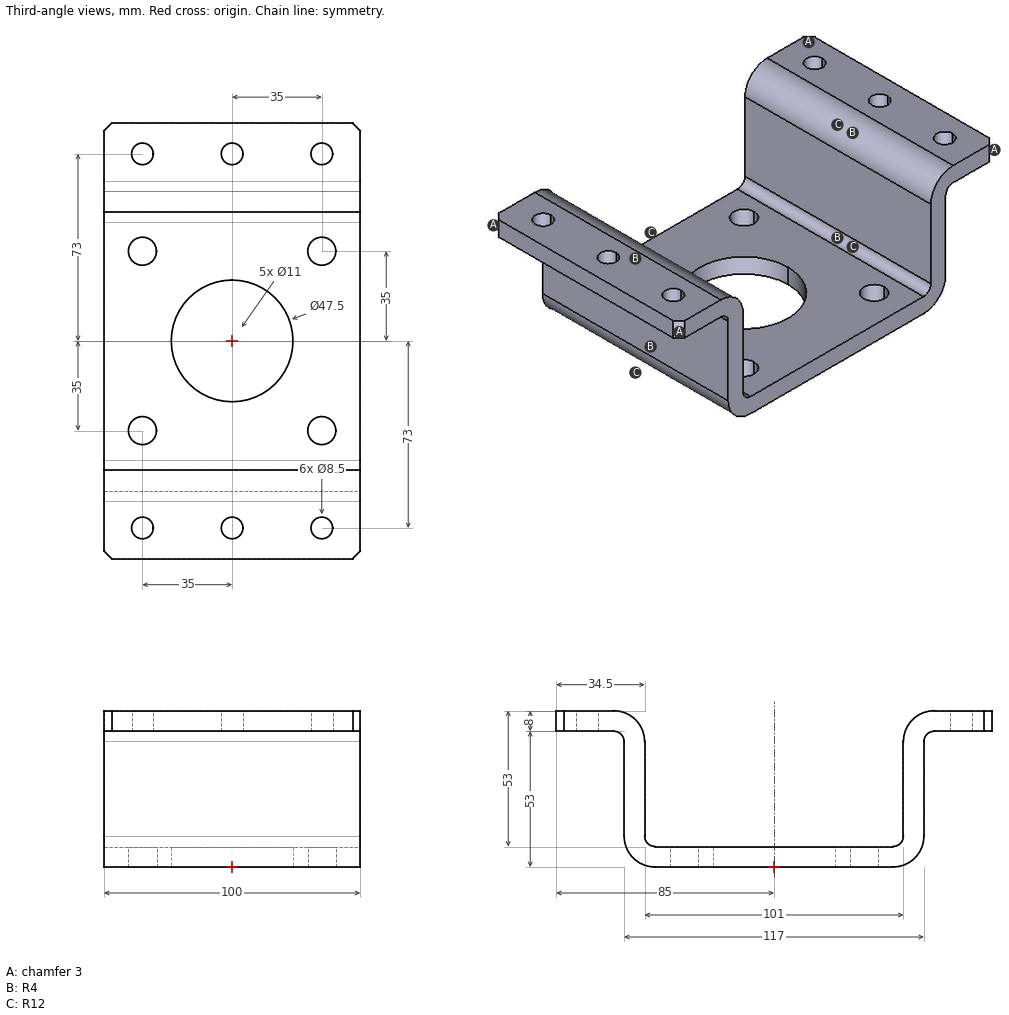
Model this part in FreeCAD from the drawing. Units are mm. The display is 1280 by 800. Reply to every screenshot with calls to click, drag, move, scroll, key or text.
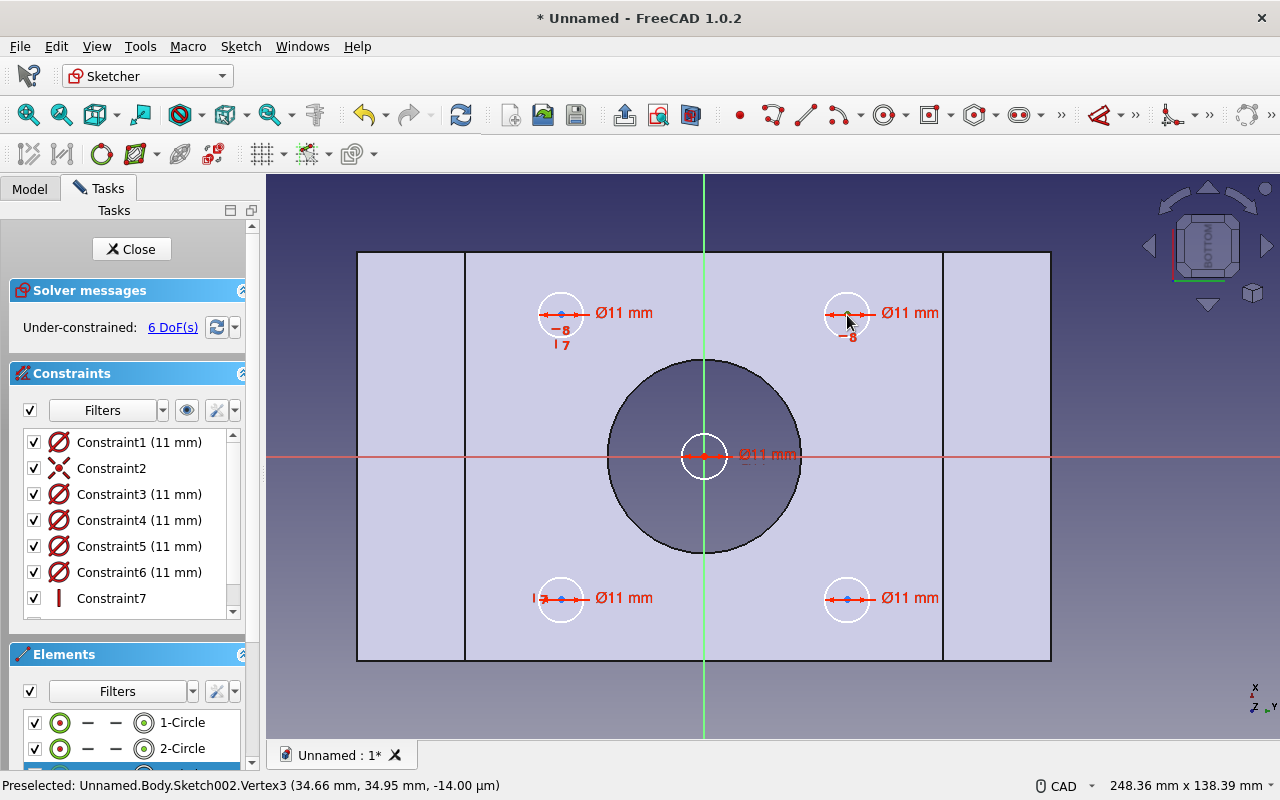
click(847, 600)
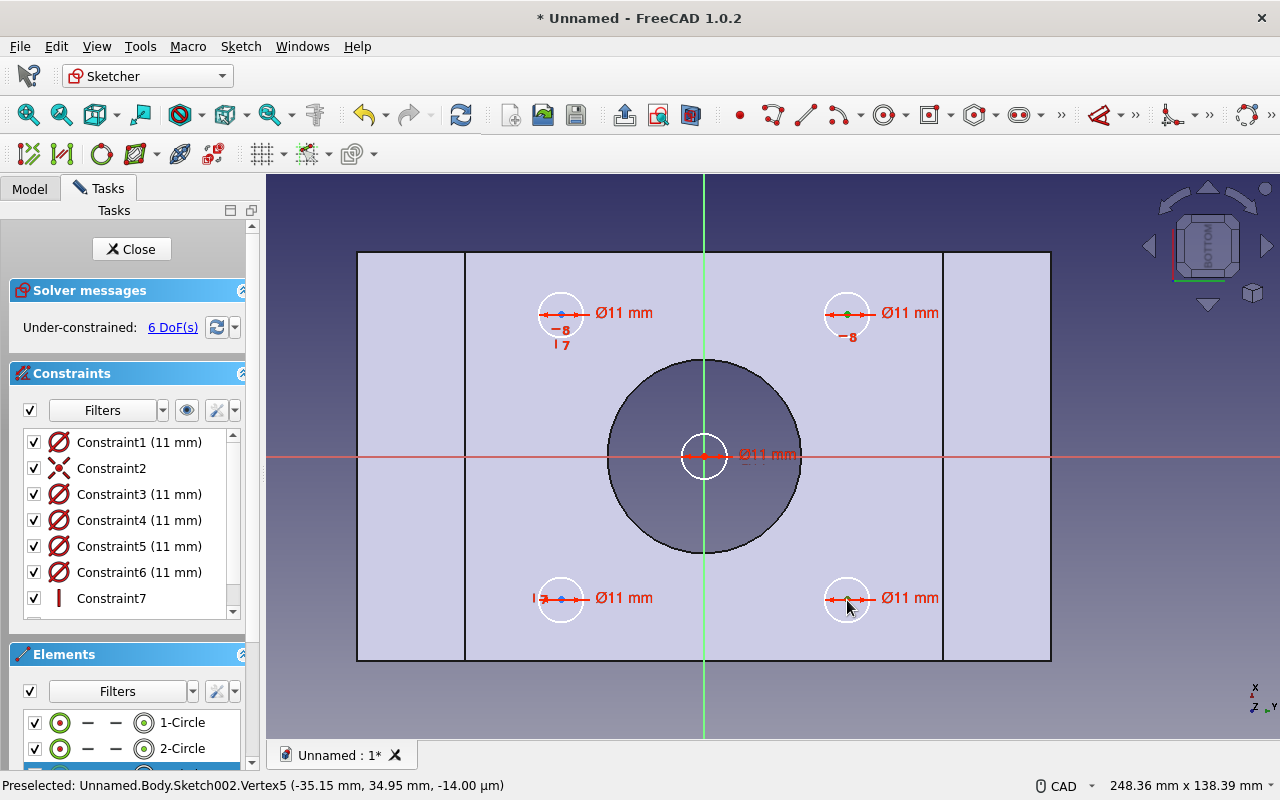
key(v)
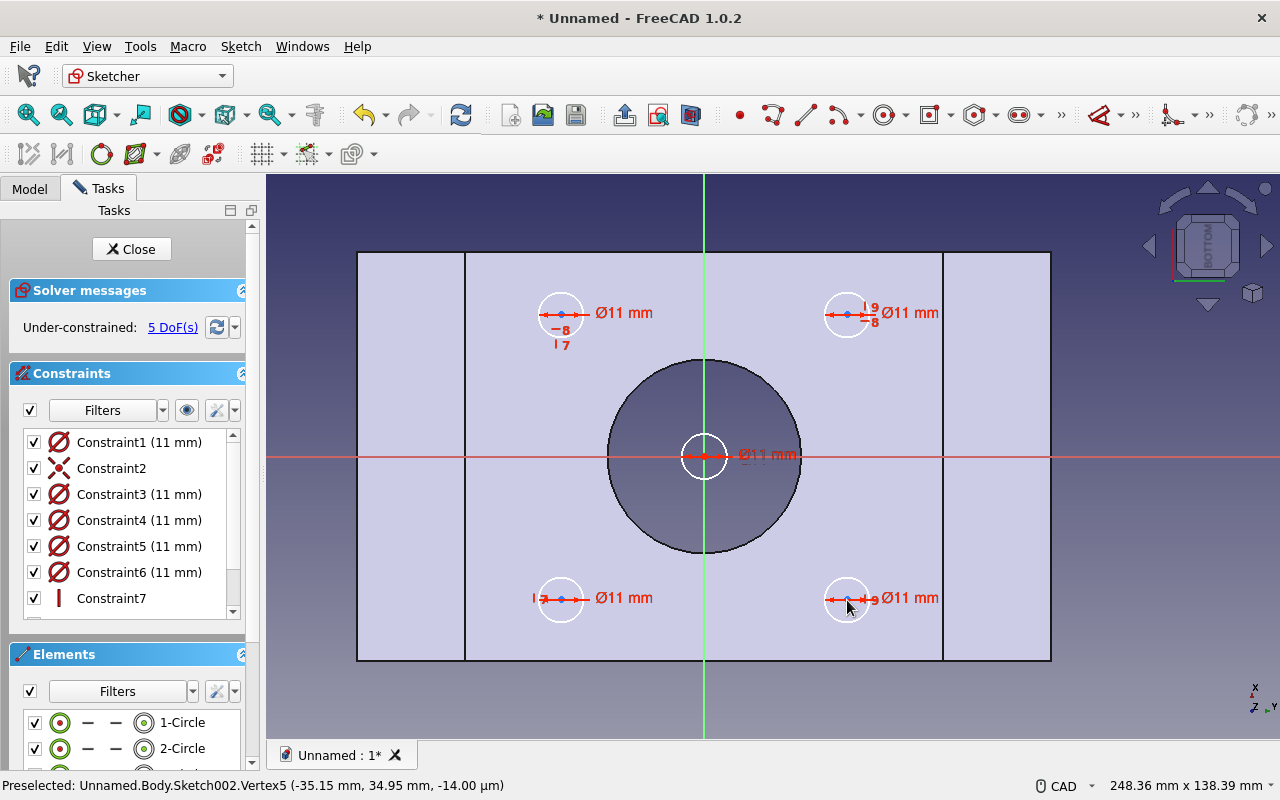
click(561, 600)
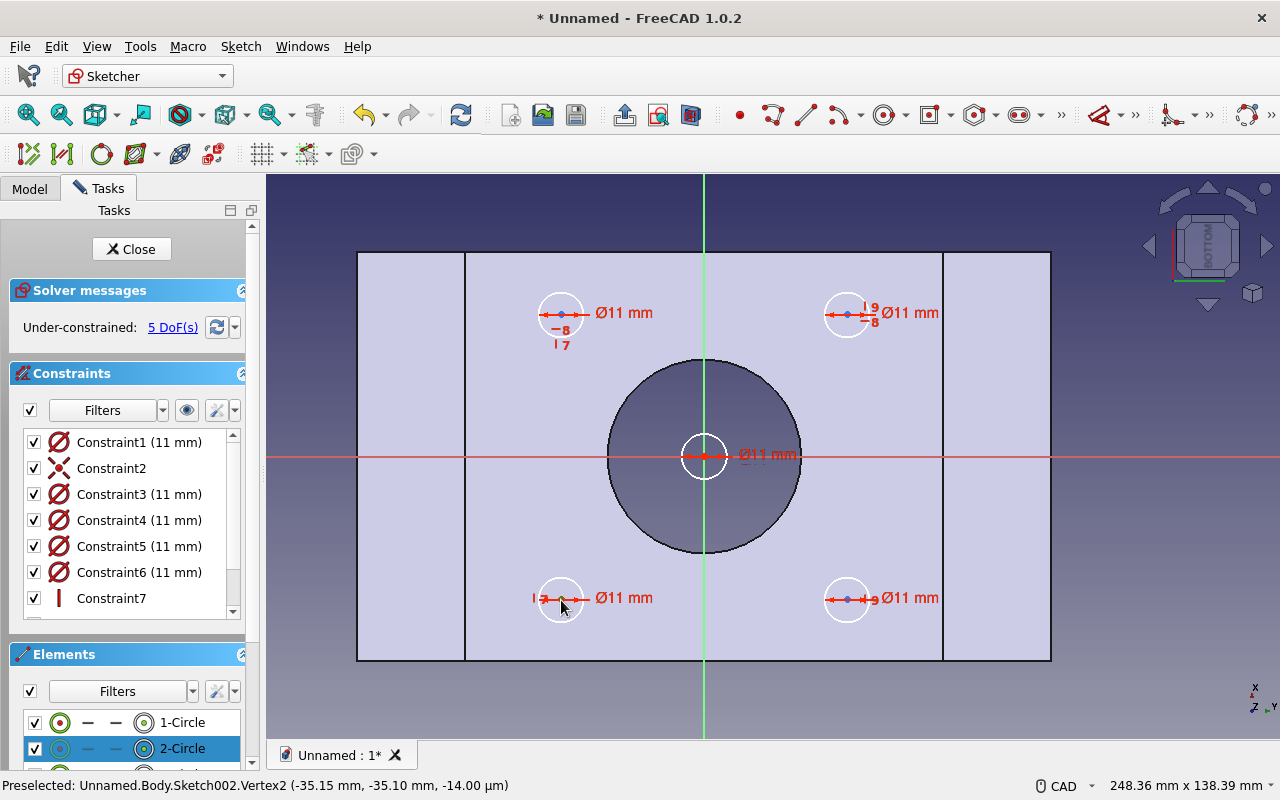
click(847, 600)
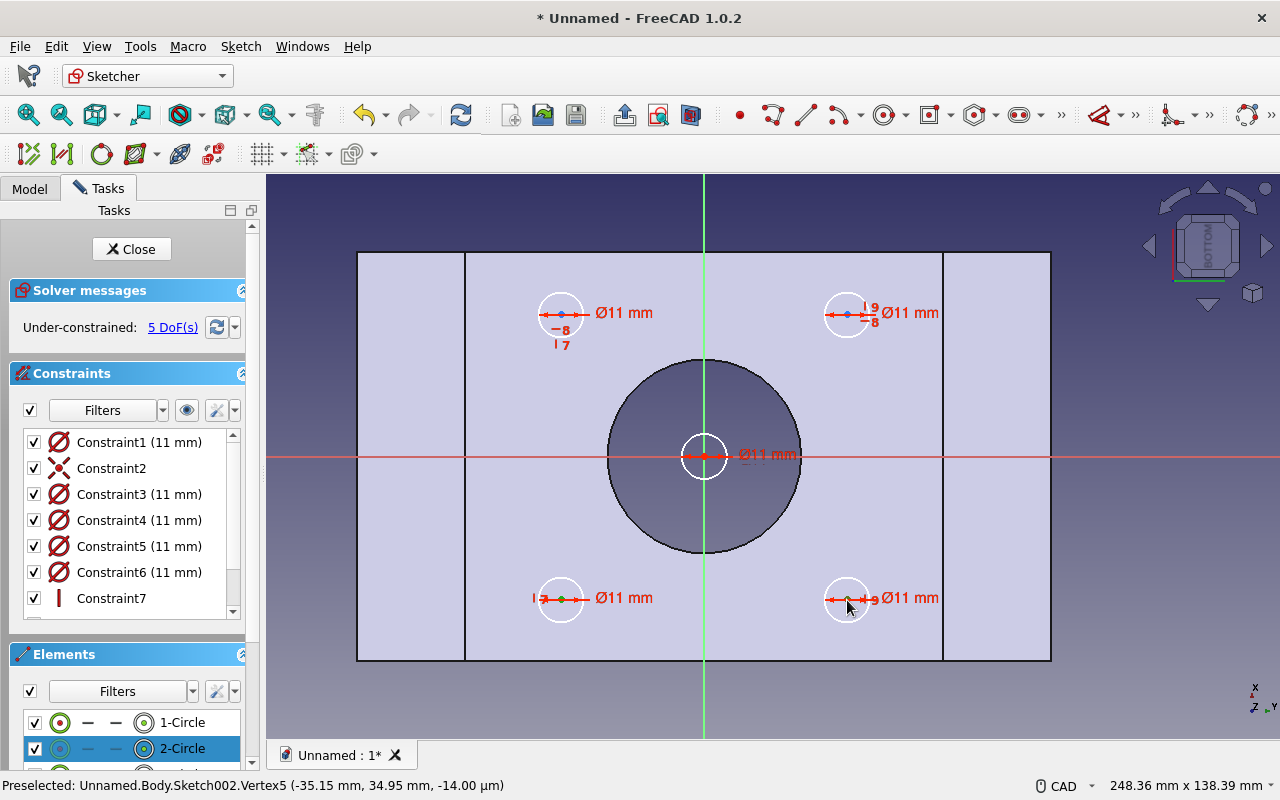
key(h)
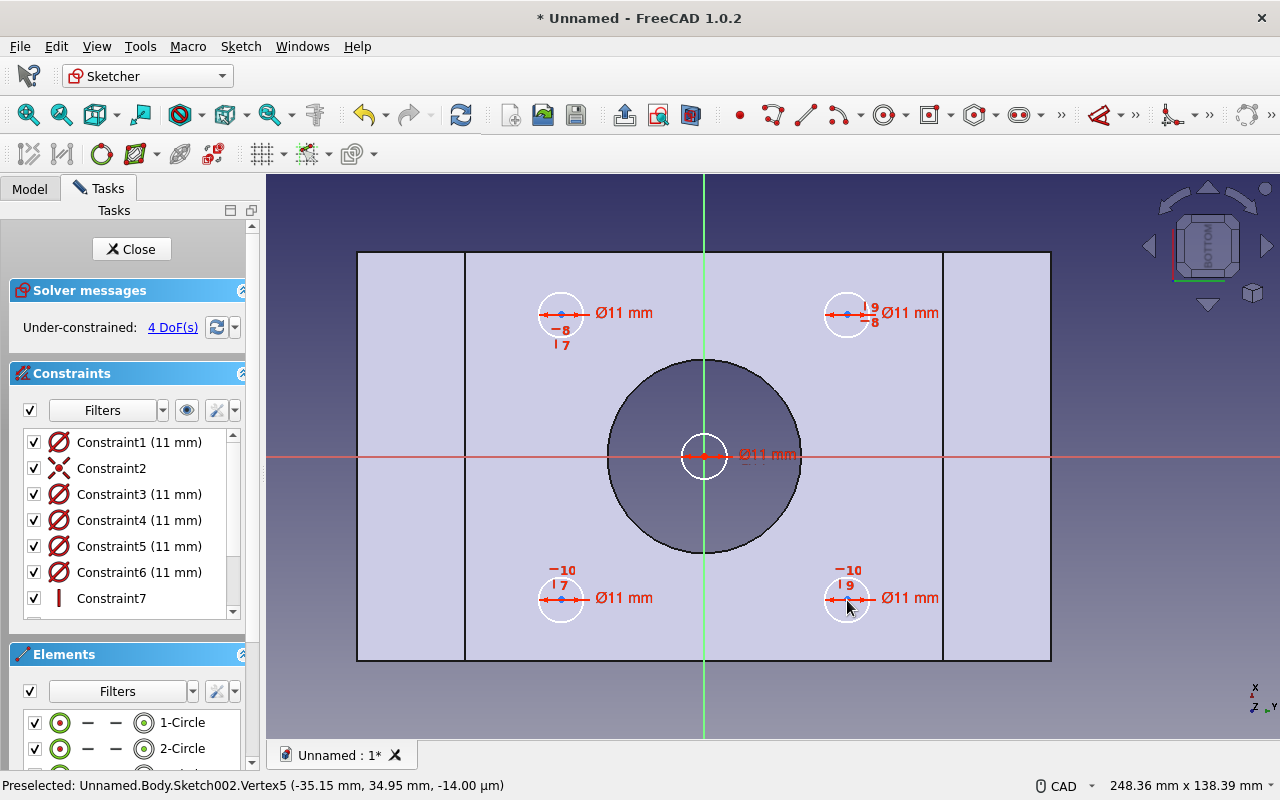
key(d)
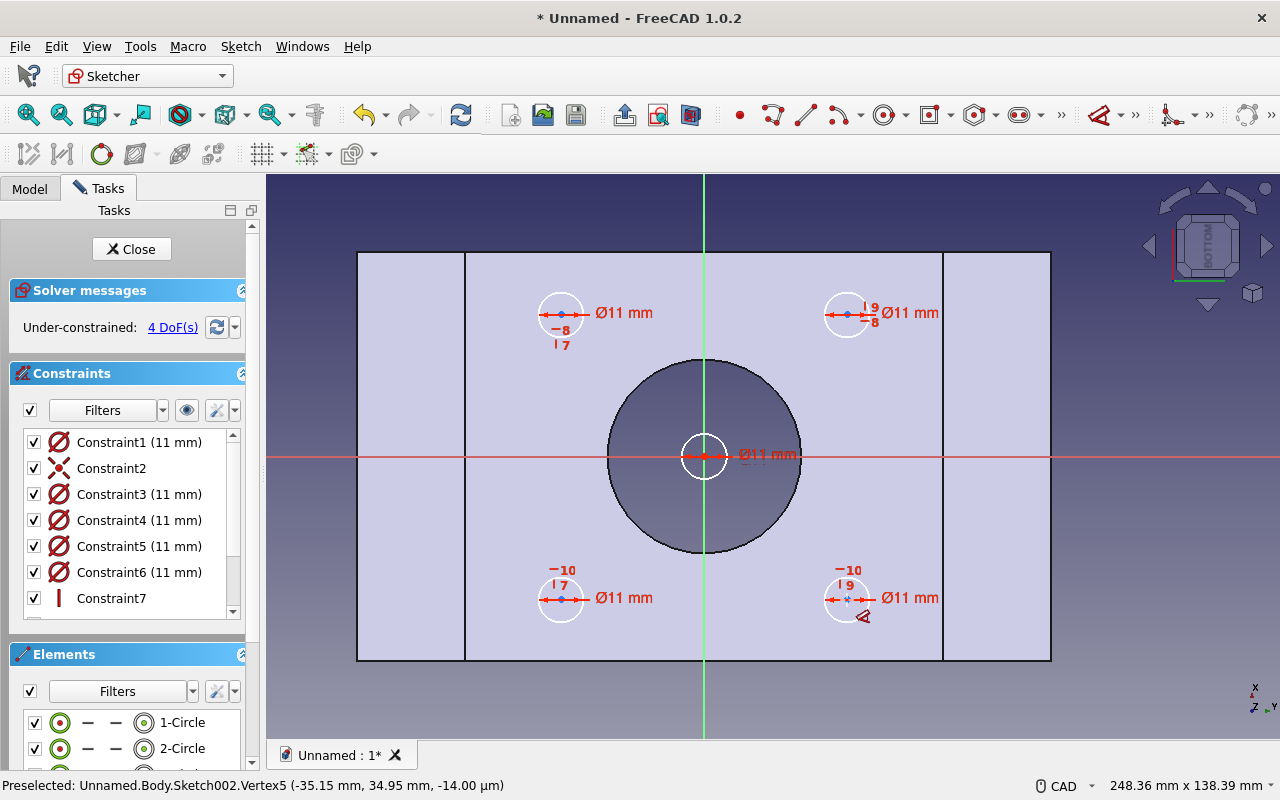
click(561, 600)
click(633, 634)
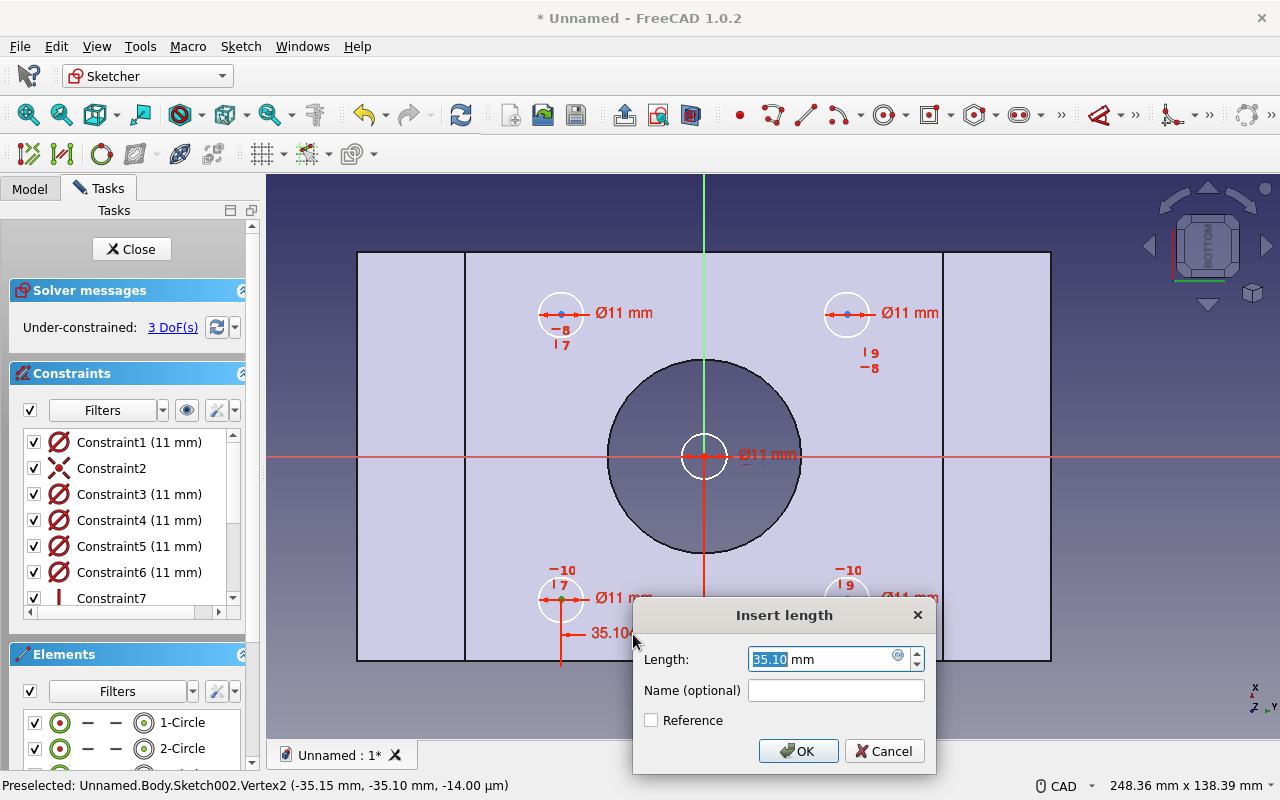
text(35)
key(Return)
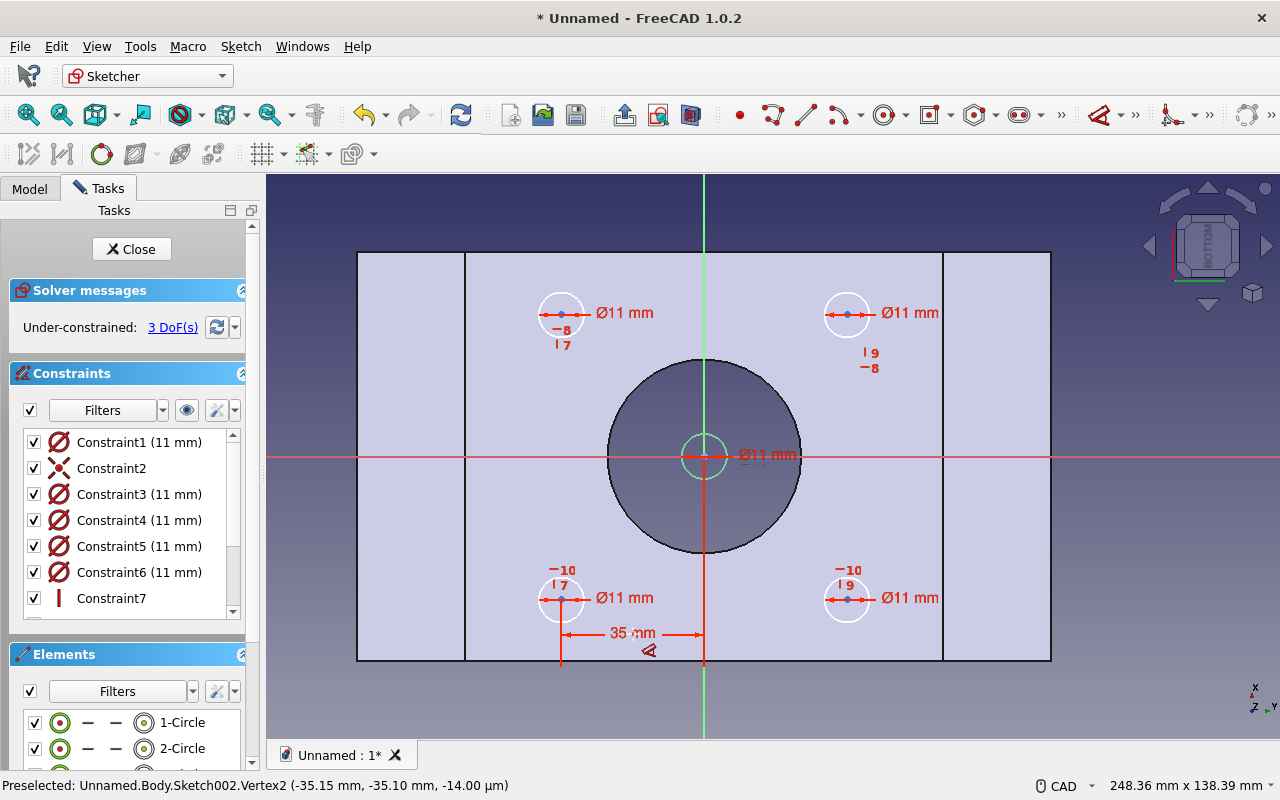
click(561, 600)
click(527, 528)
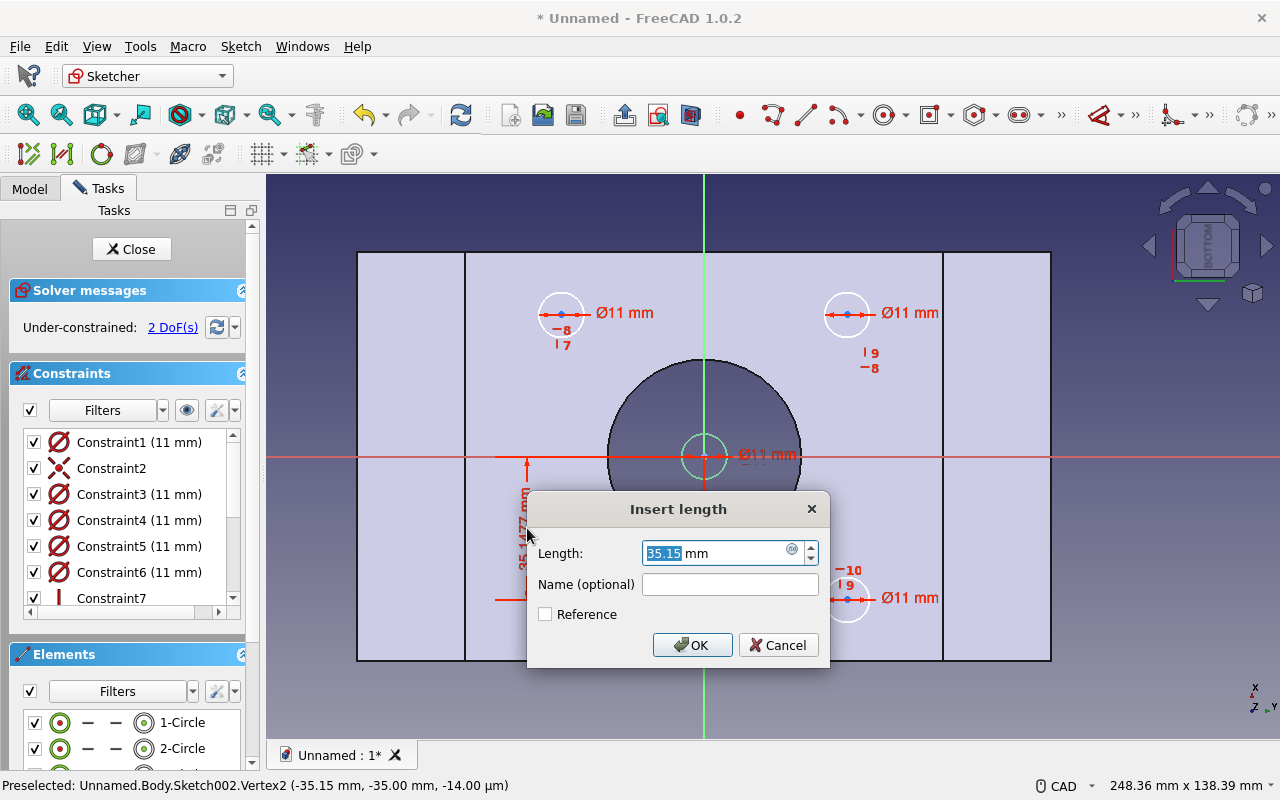
text(35)
key(Return)